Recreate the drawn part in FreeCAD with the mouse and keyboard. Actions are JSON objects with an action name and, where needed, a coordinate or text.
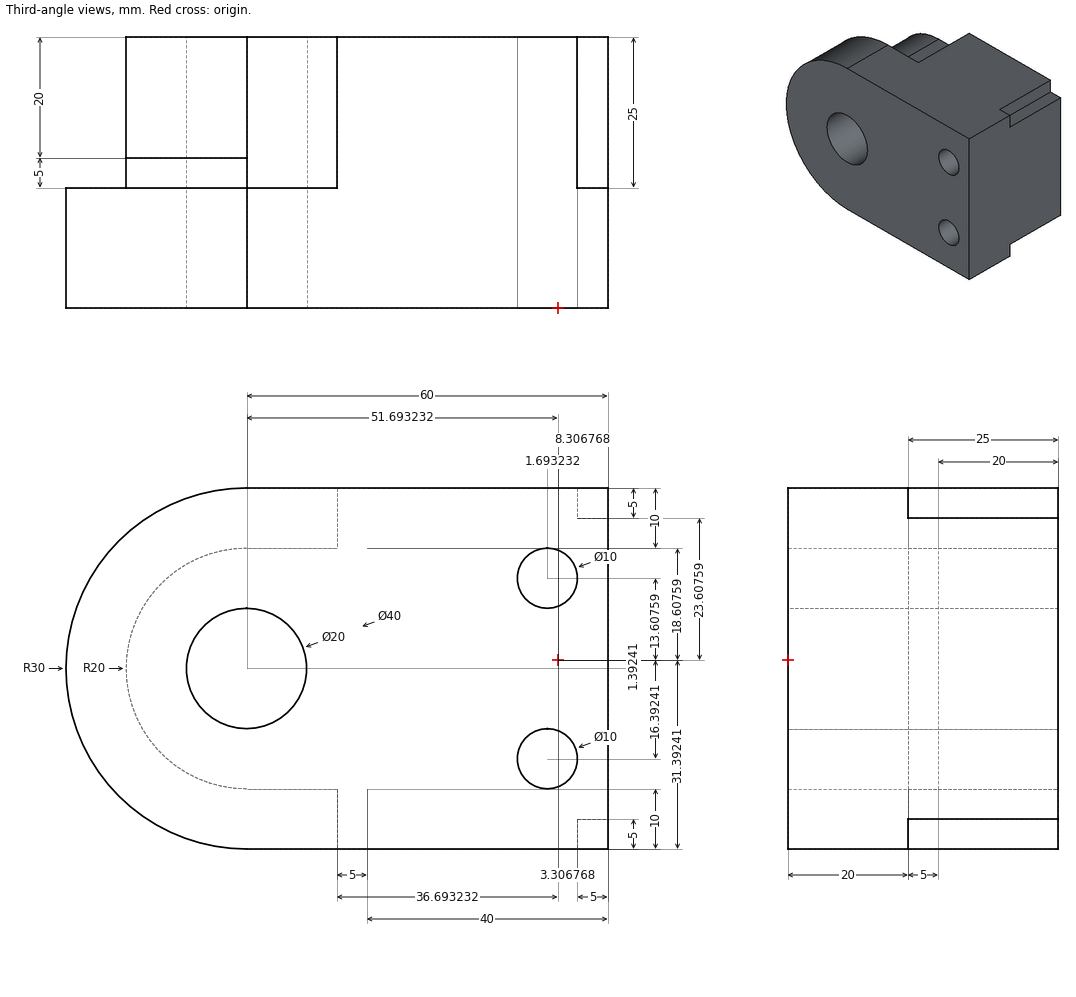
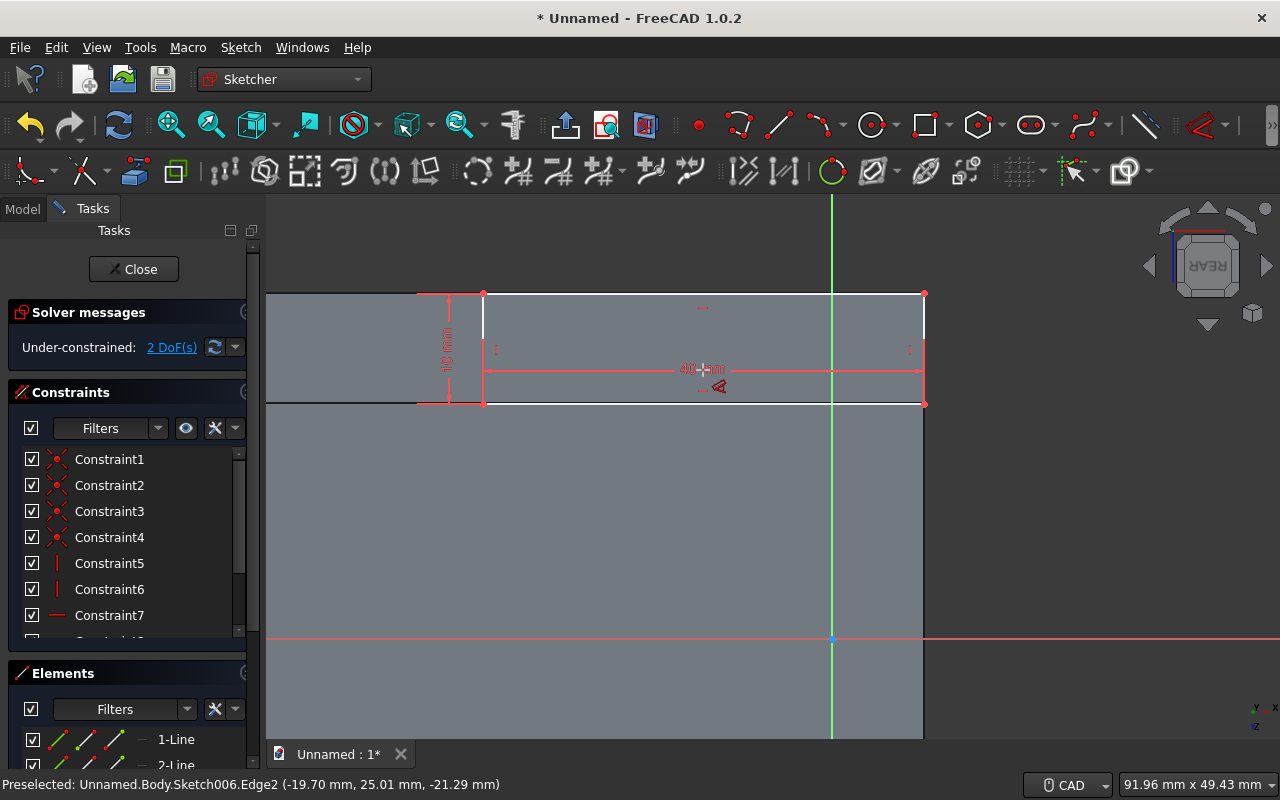
{"action": "left_click", "coordinate": [483, 294]}
{"action": "left_click", "coordinate": [449, 467]}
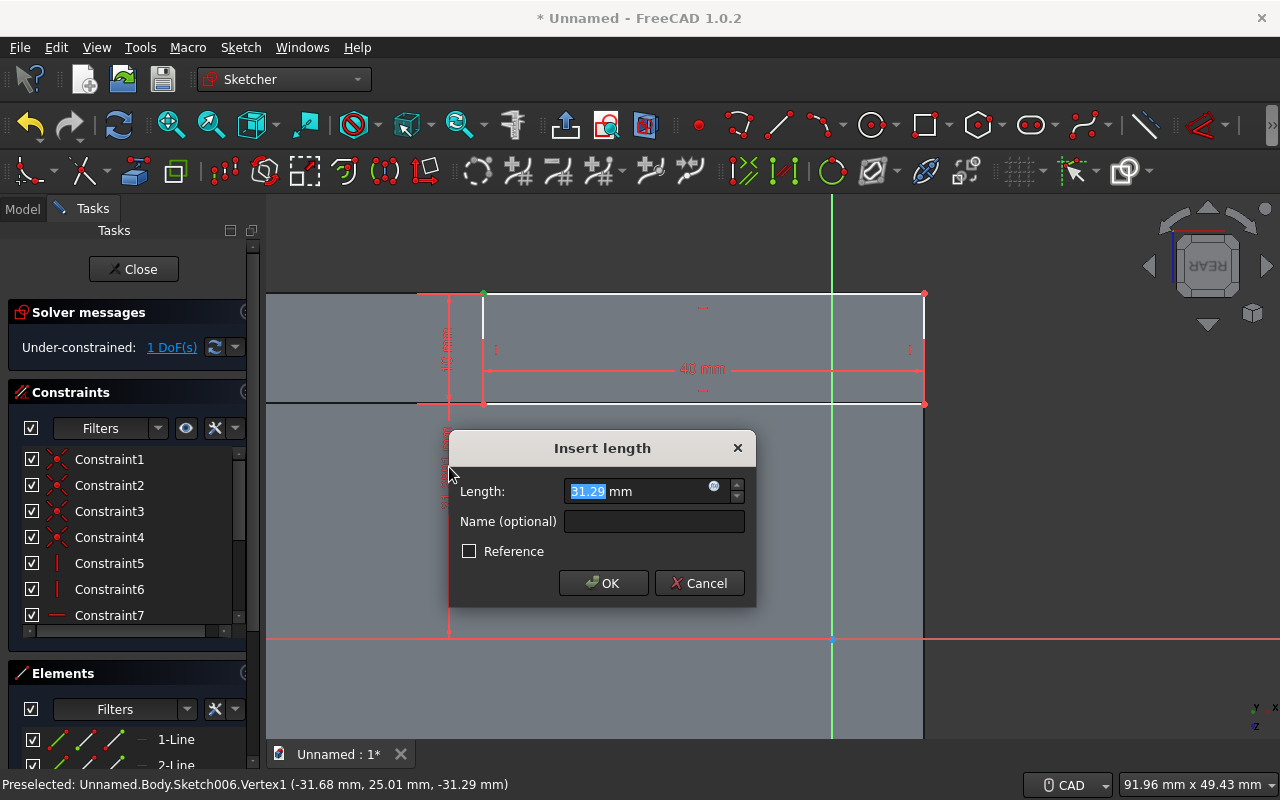
{"action": "type", "text": "31.39241"}
{"action": "key", "text": "Return"}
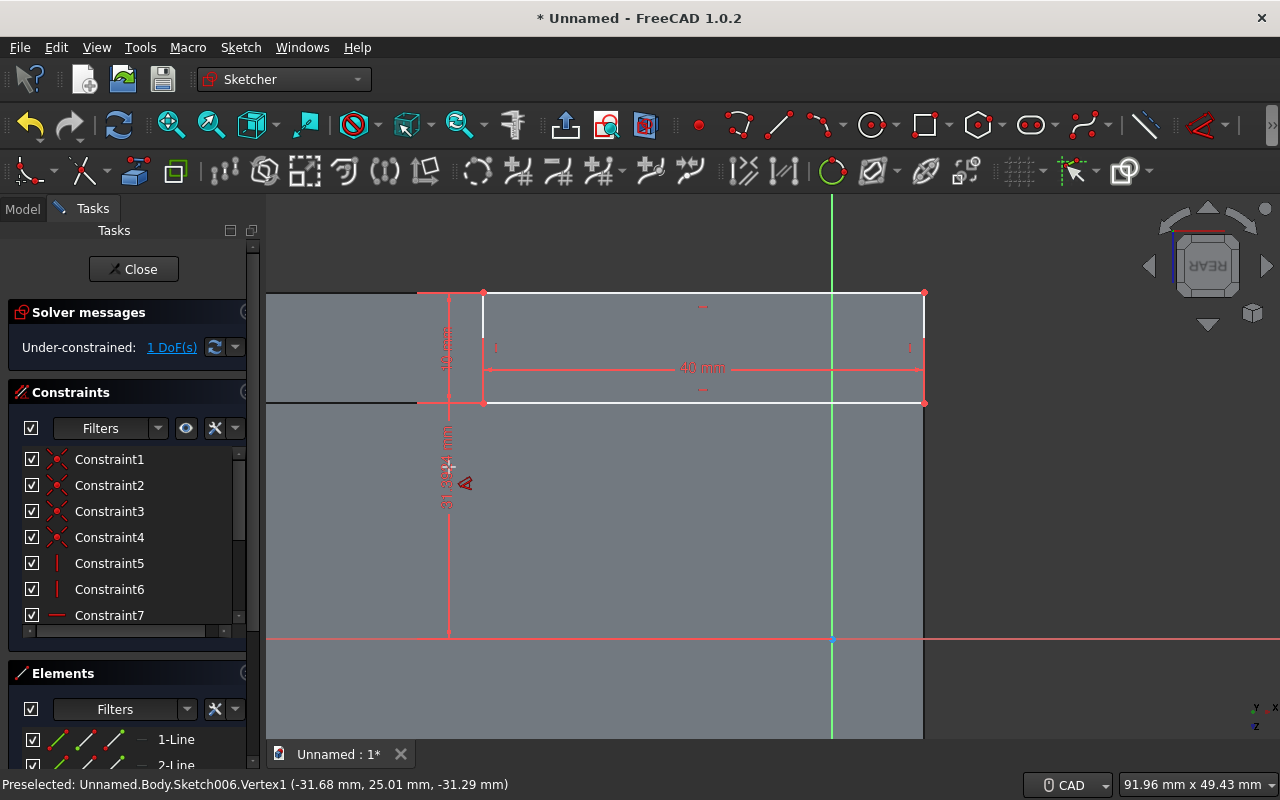
{"action": "left_click", "coordinate": [924, 403]}
{"action": "left_click", "coordinate": [878, 673]}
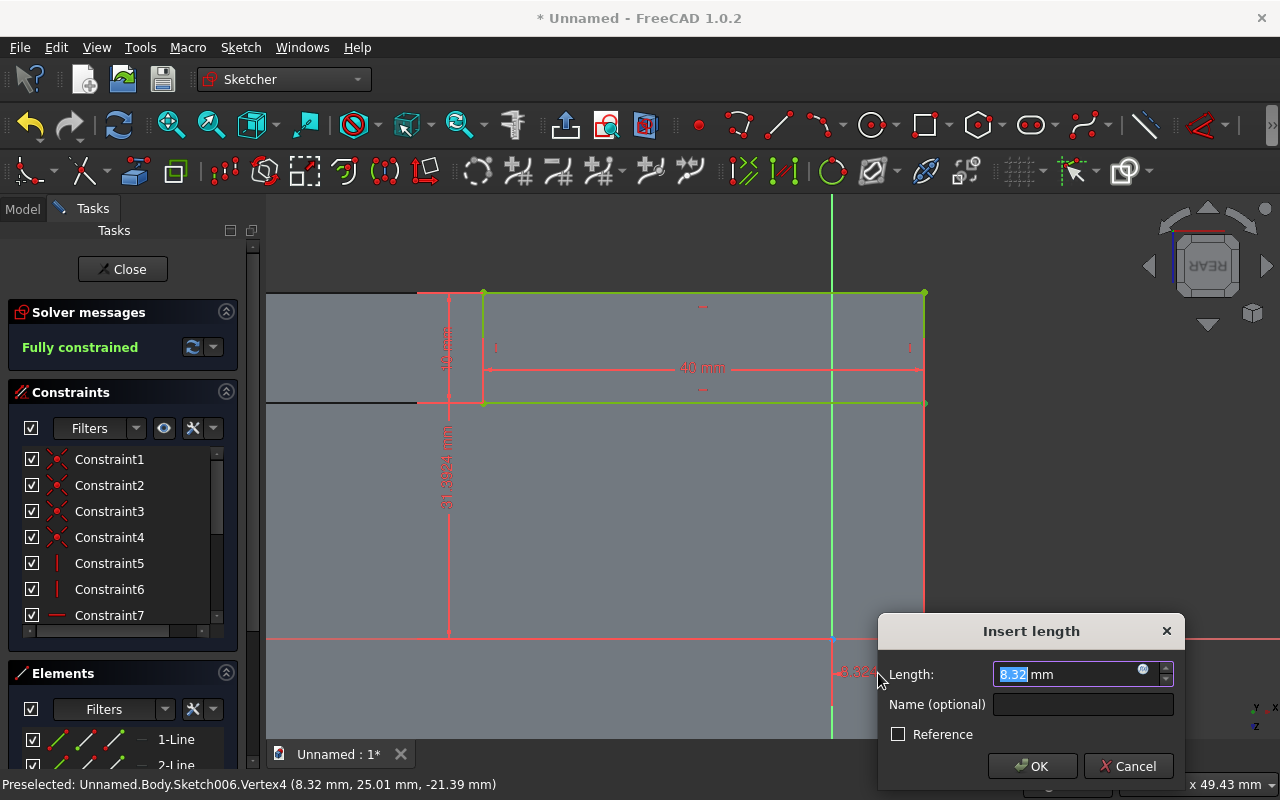
{"action": "type", "text": "8.306768"}
{"action": "key", "text": "Return"}
{"action": "key", "text": "Escape"}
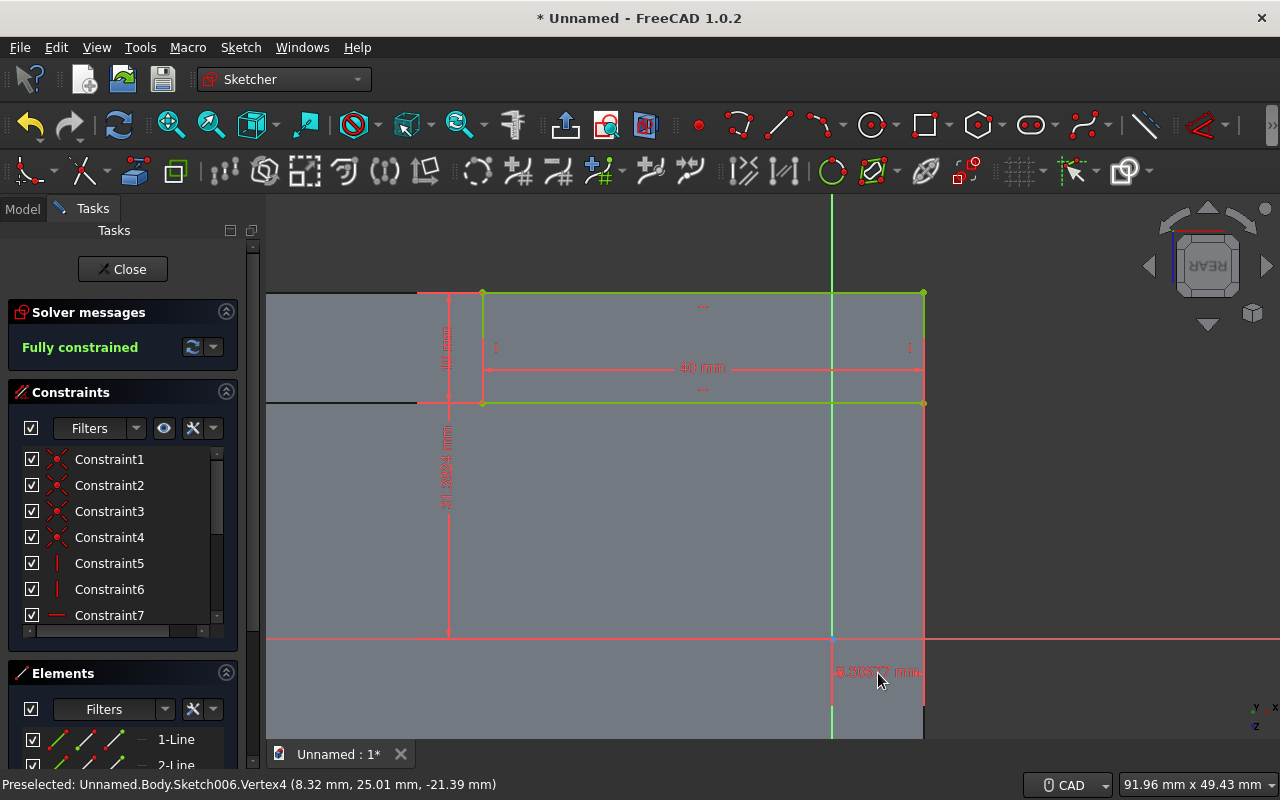
{"action": "left_click", "coordinate": [123, 269]}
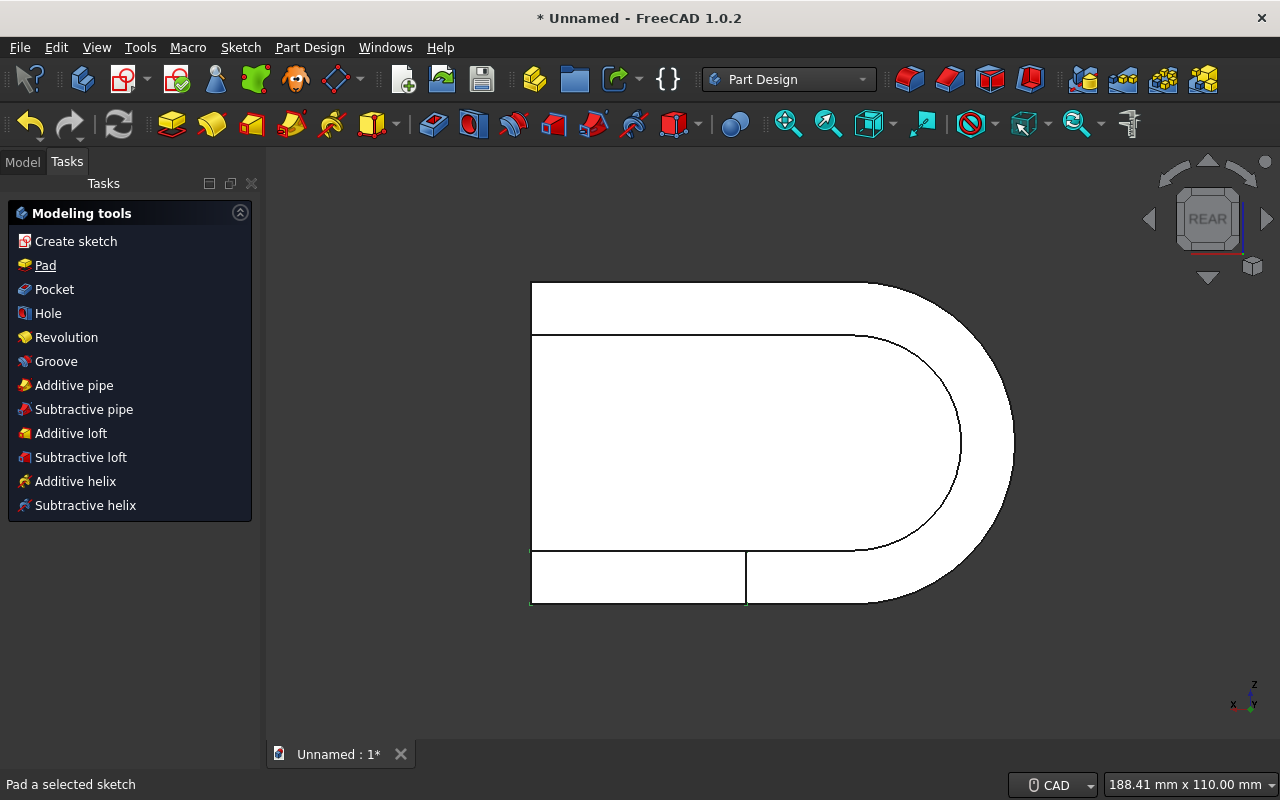
{"action": "left_click", "coordinate": [172, 124]}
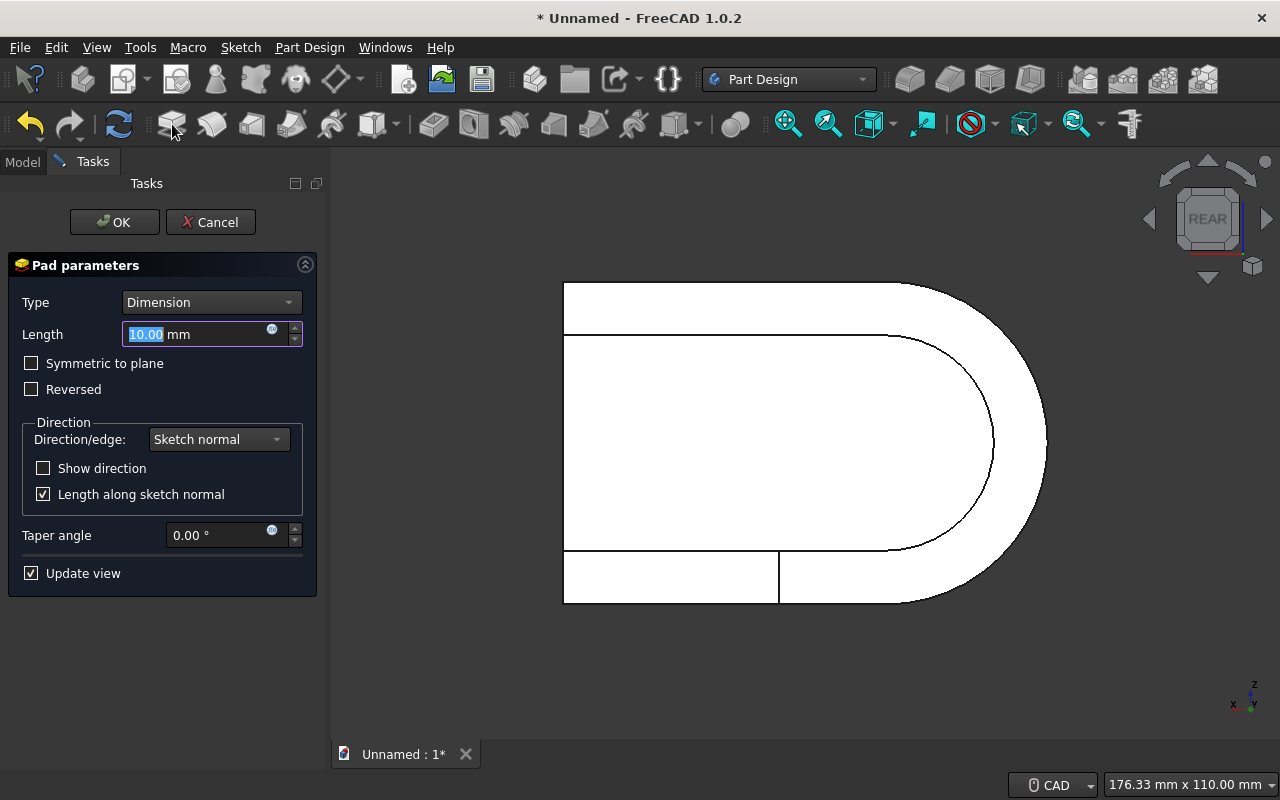
{"action": "type", "text": "20"}
{"action": "key", "text": "Tab"}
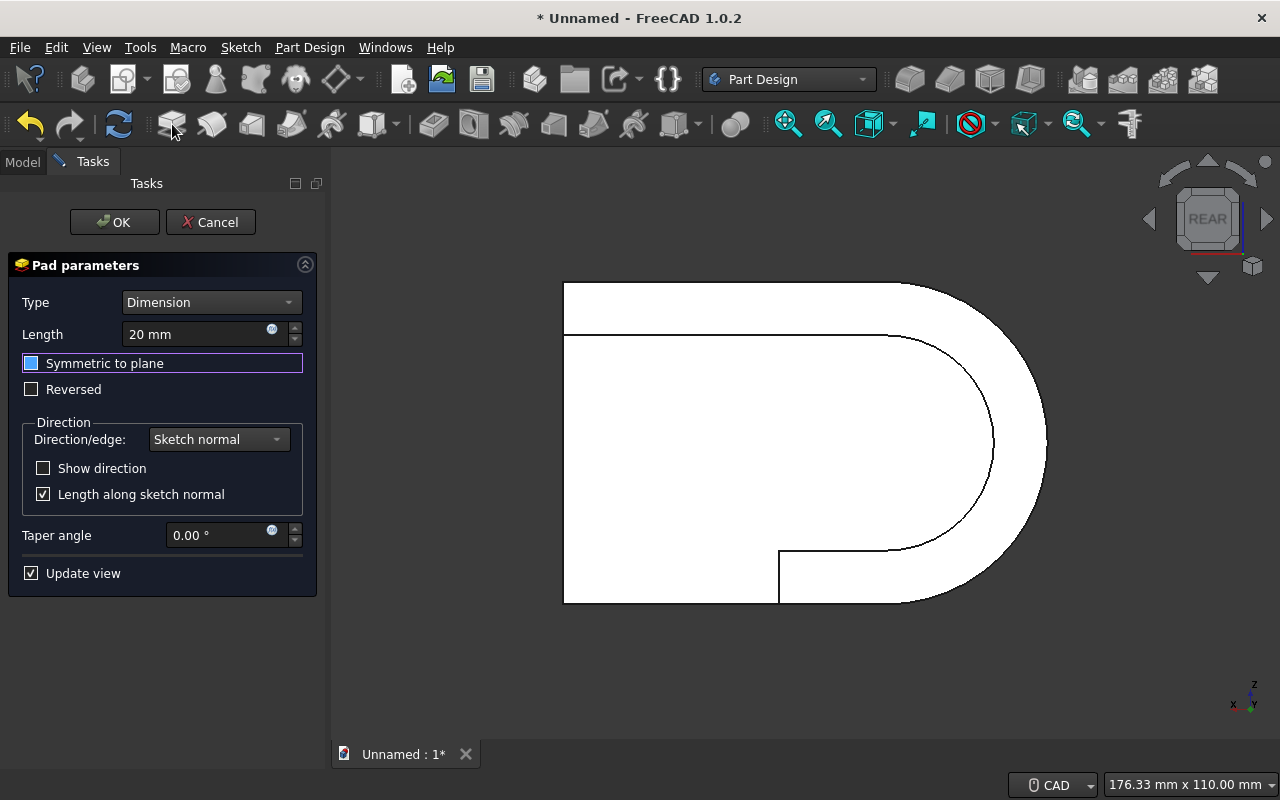
{"action": "left_click", "coordinate": [115, 222]}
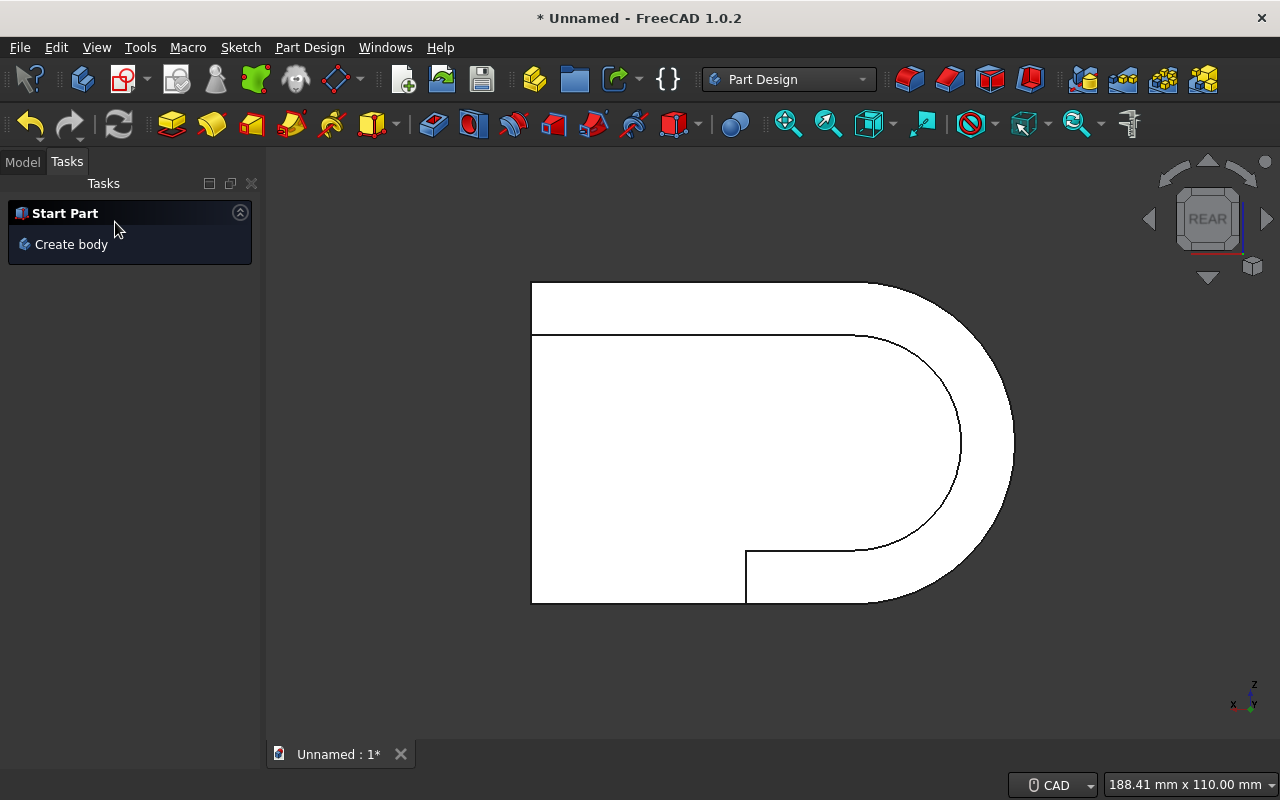
{"action": "left_click", "coordinate": [981, 488]}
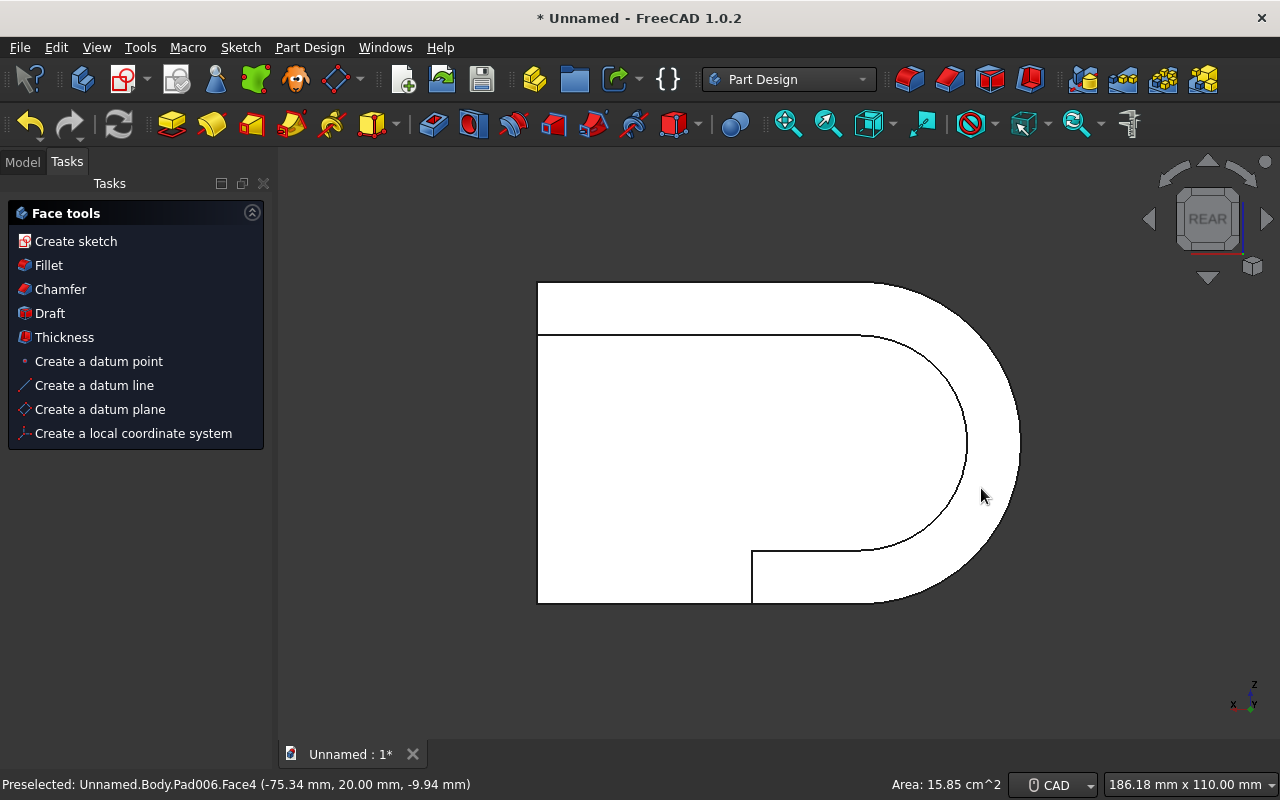
{"action": "left_click", "coordinate": [124, 80]}